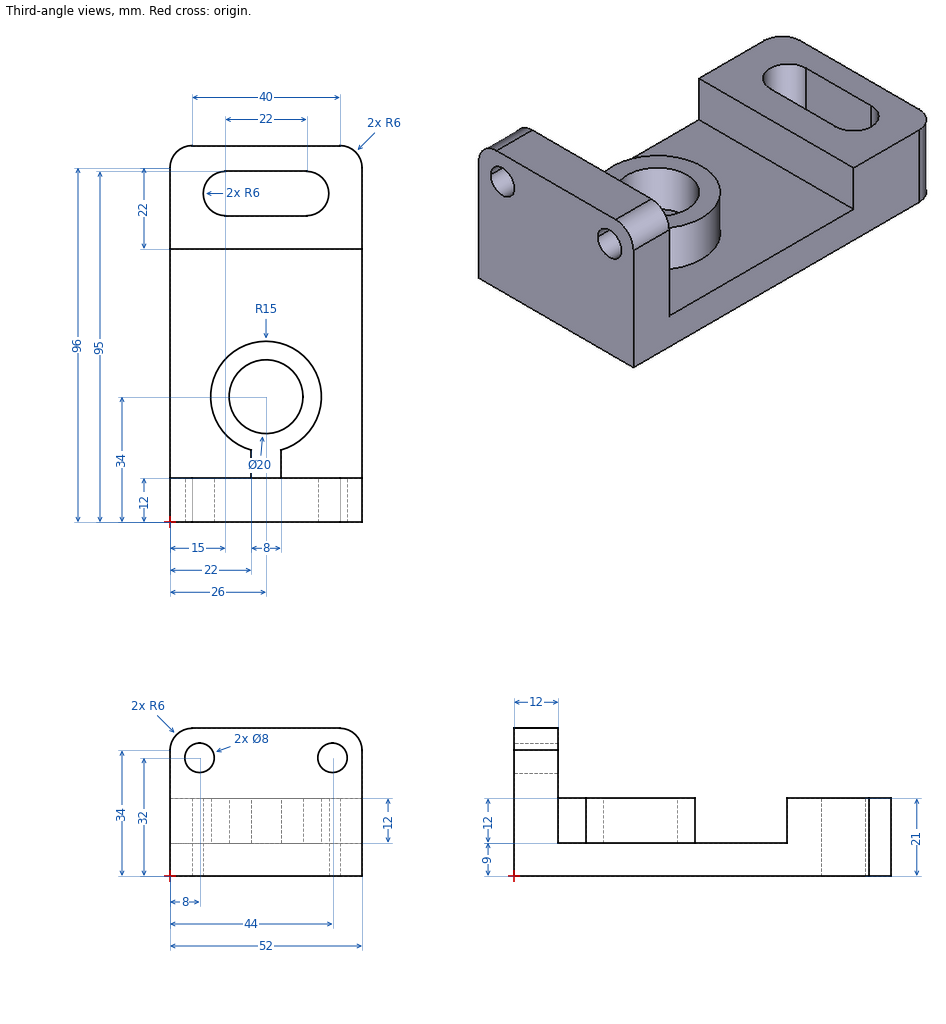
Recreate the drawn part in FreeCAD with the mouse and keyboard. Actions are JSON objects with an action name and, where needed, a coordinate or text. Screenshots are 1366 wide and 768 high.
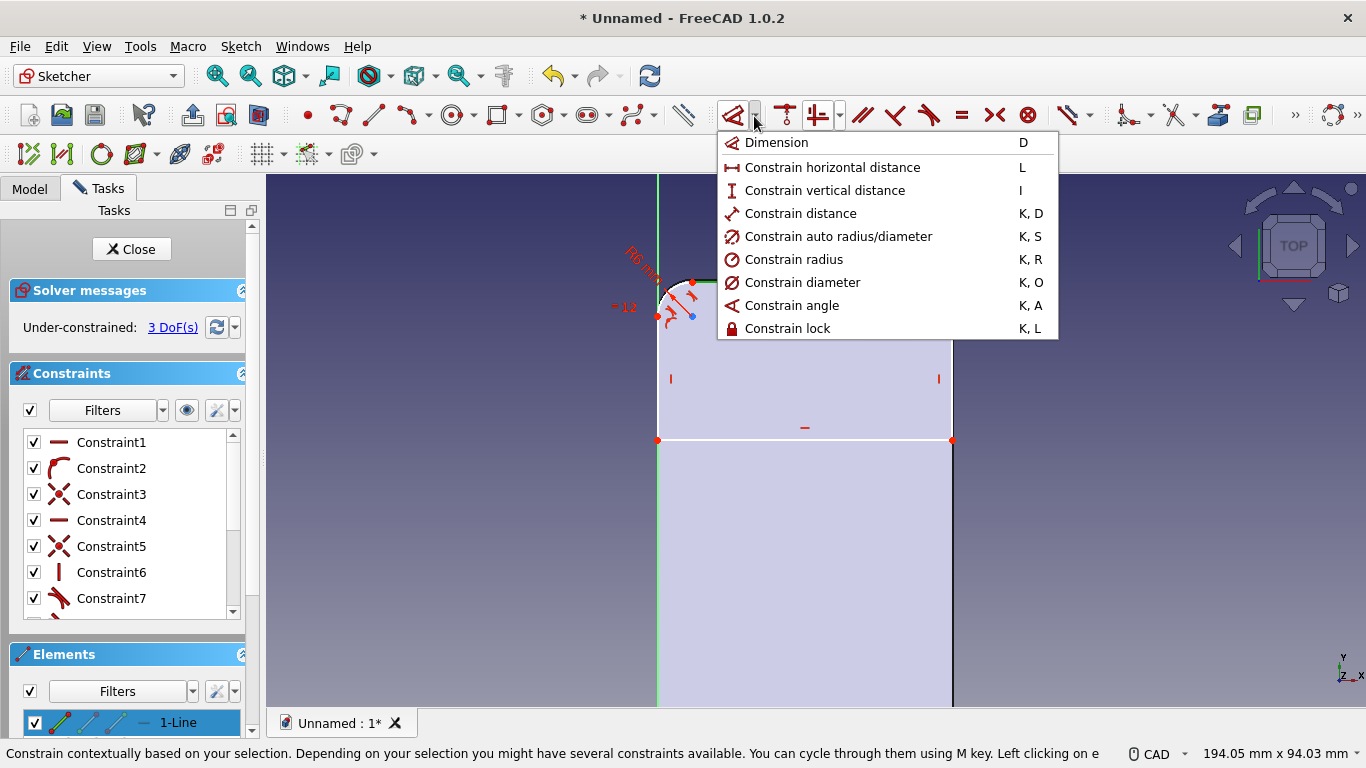
{"action": "left_click", "coordinate": [888, 168]}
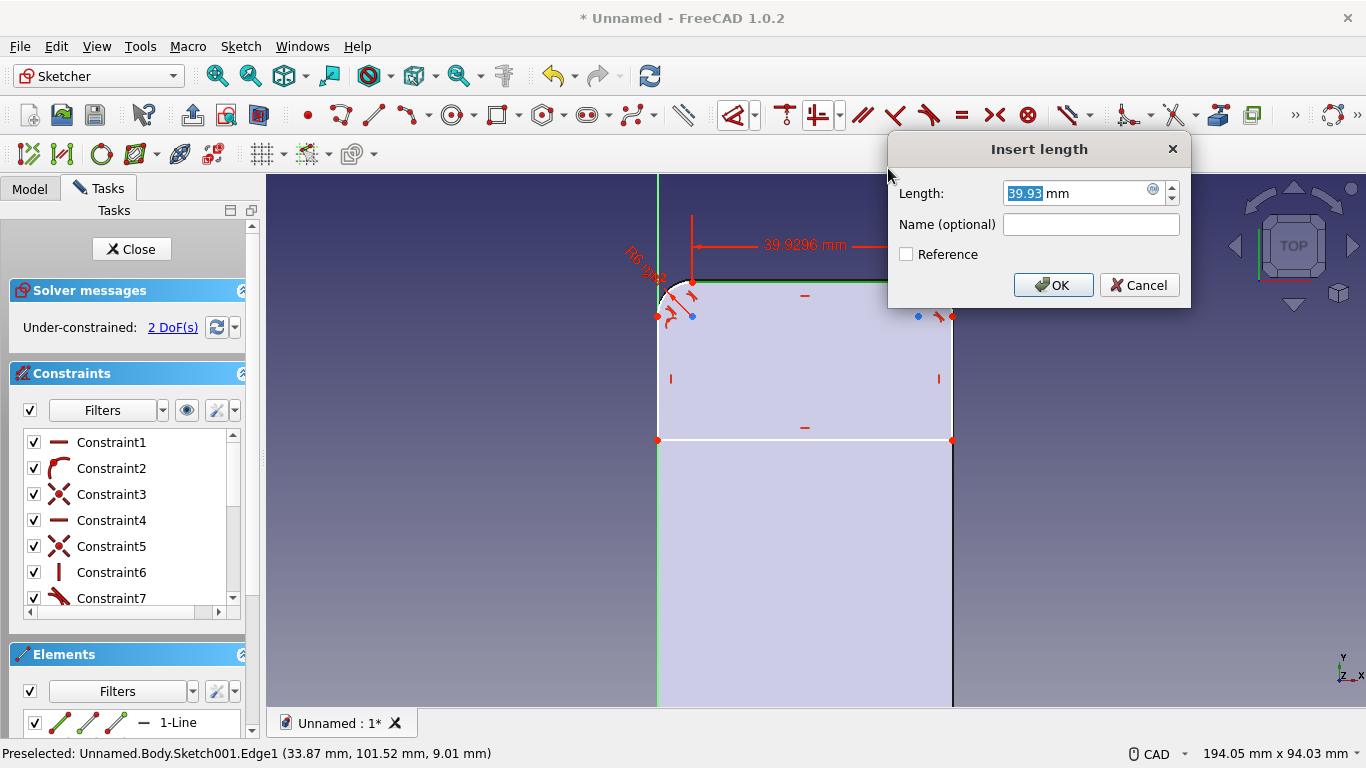
{"action": "type", "text": "40"}
{"action": "key", "text": "Return"}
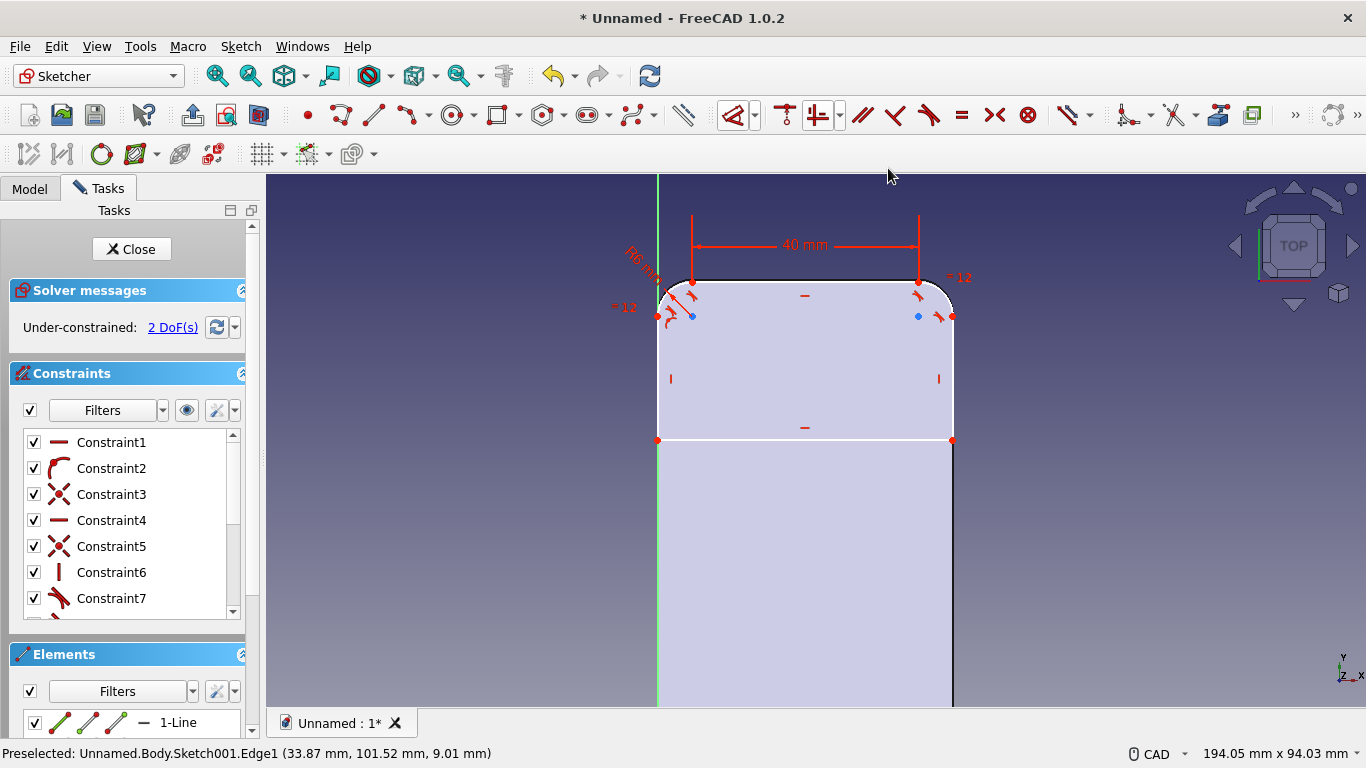
{"action": "left_click", "coordinate": [658, 354]}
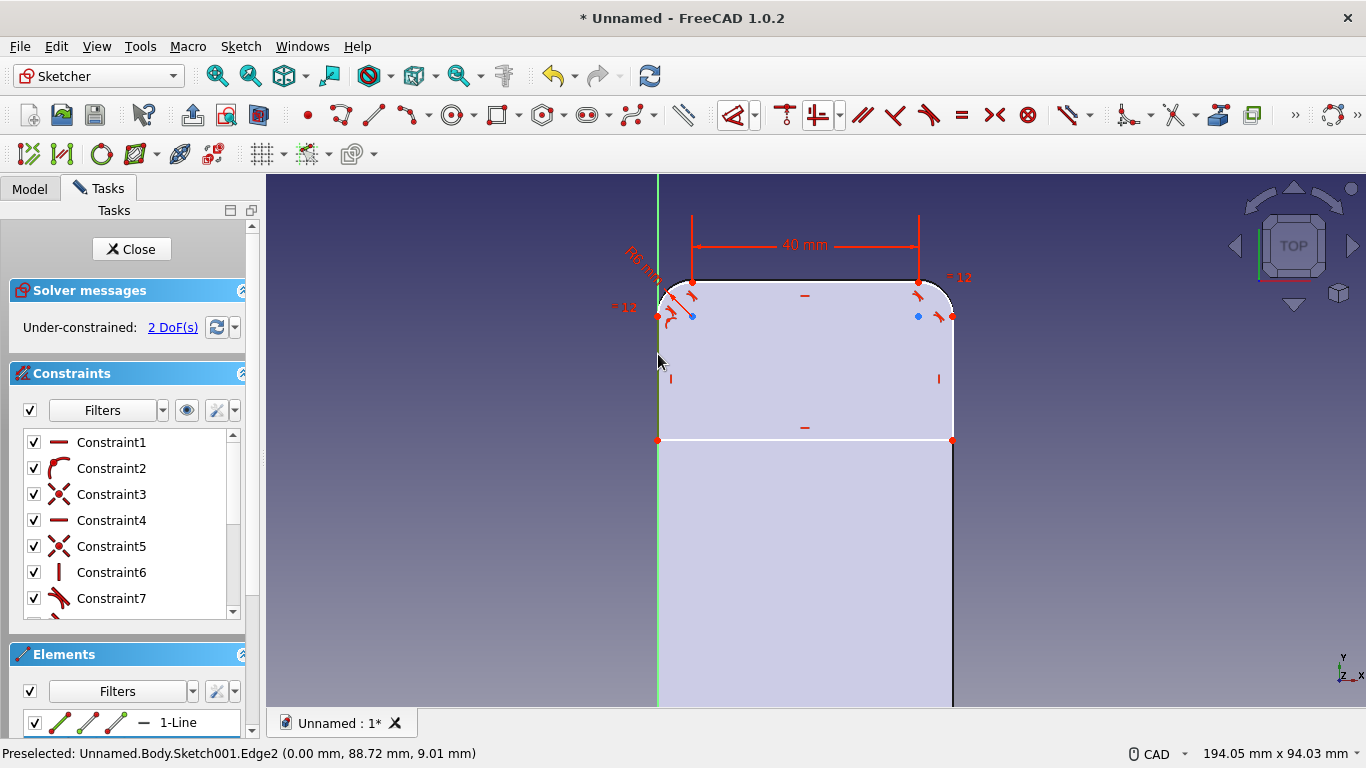
{"action": "key", "text": "i"}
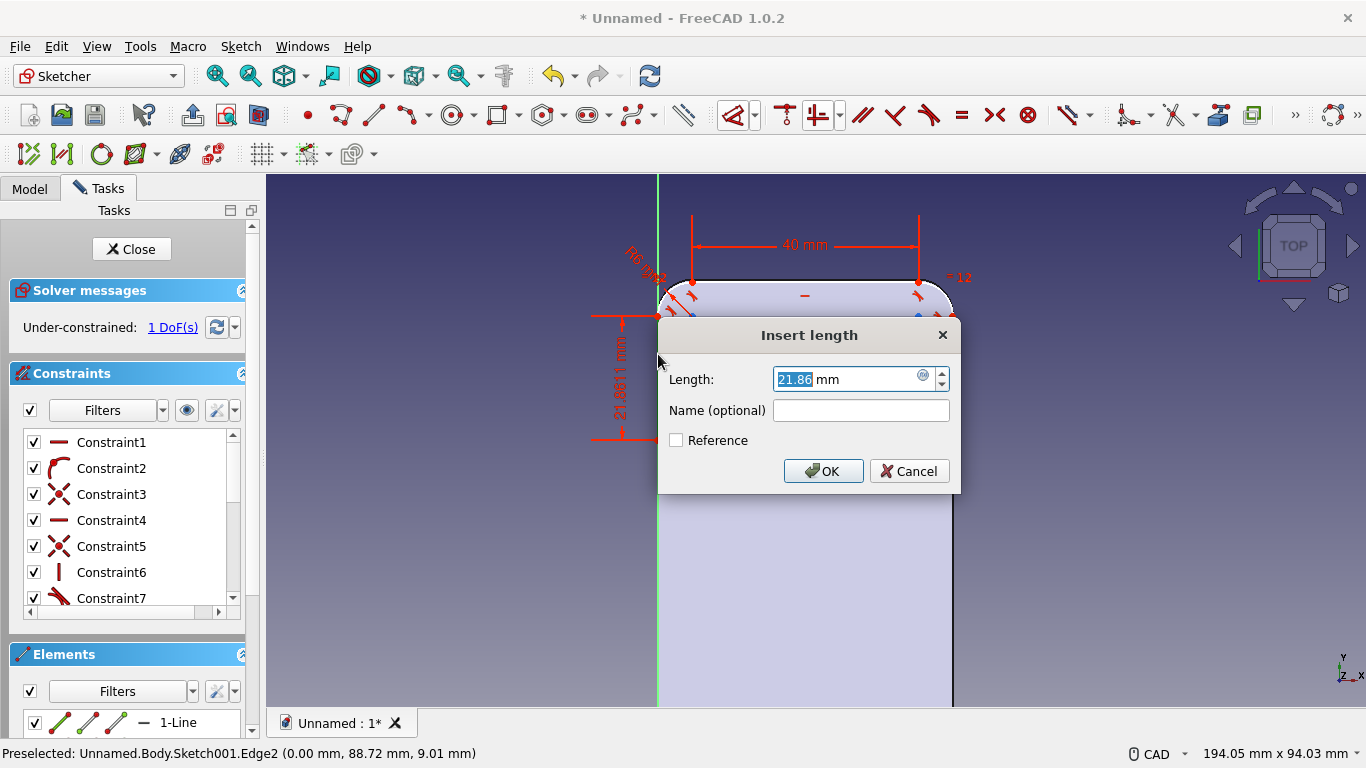
{"action": "type", "text": "22"}
{"action": "key", "text": "Return"}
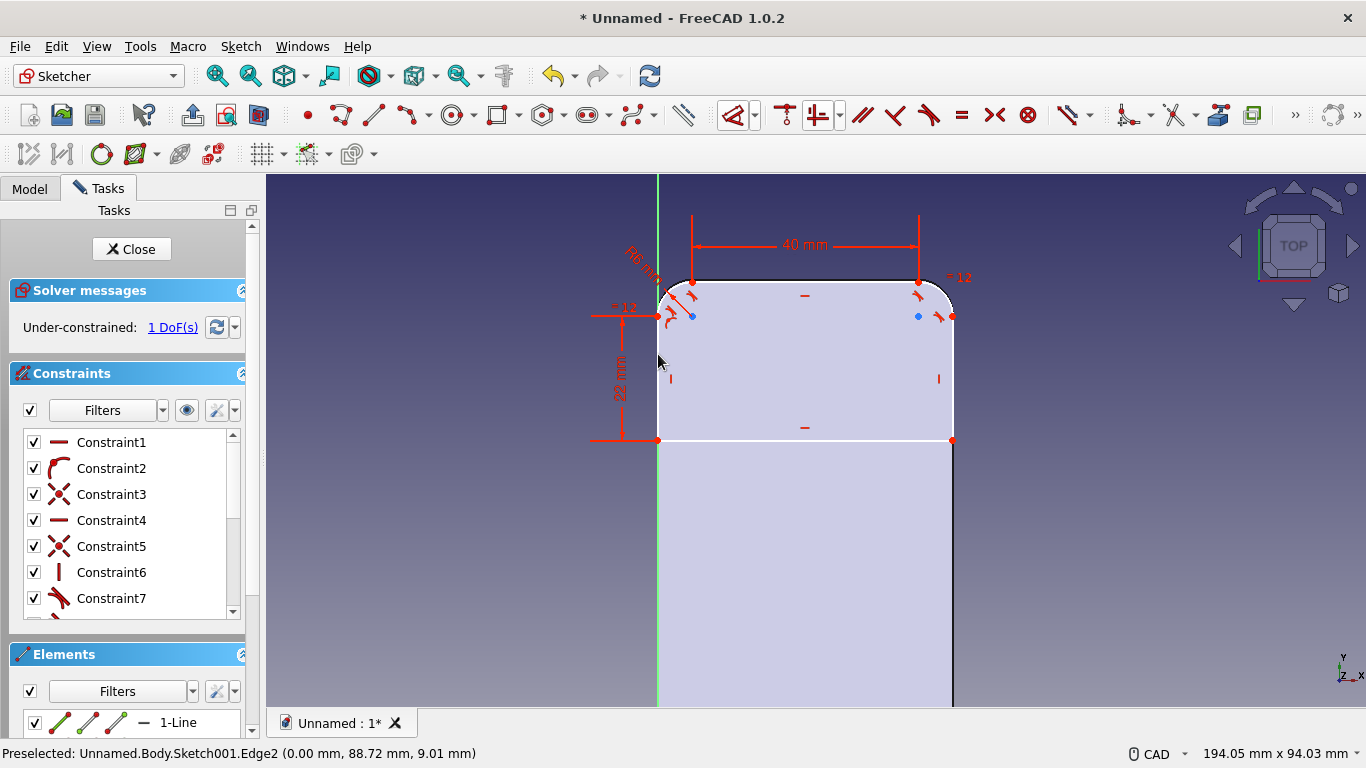
{"action": "left_click", "coordinate": [658, 316]}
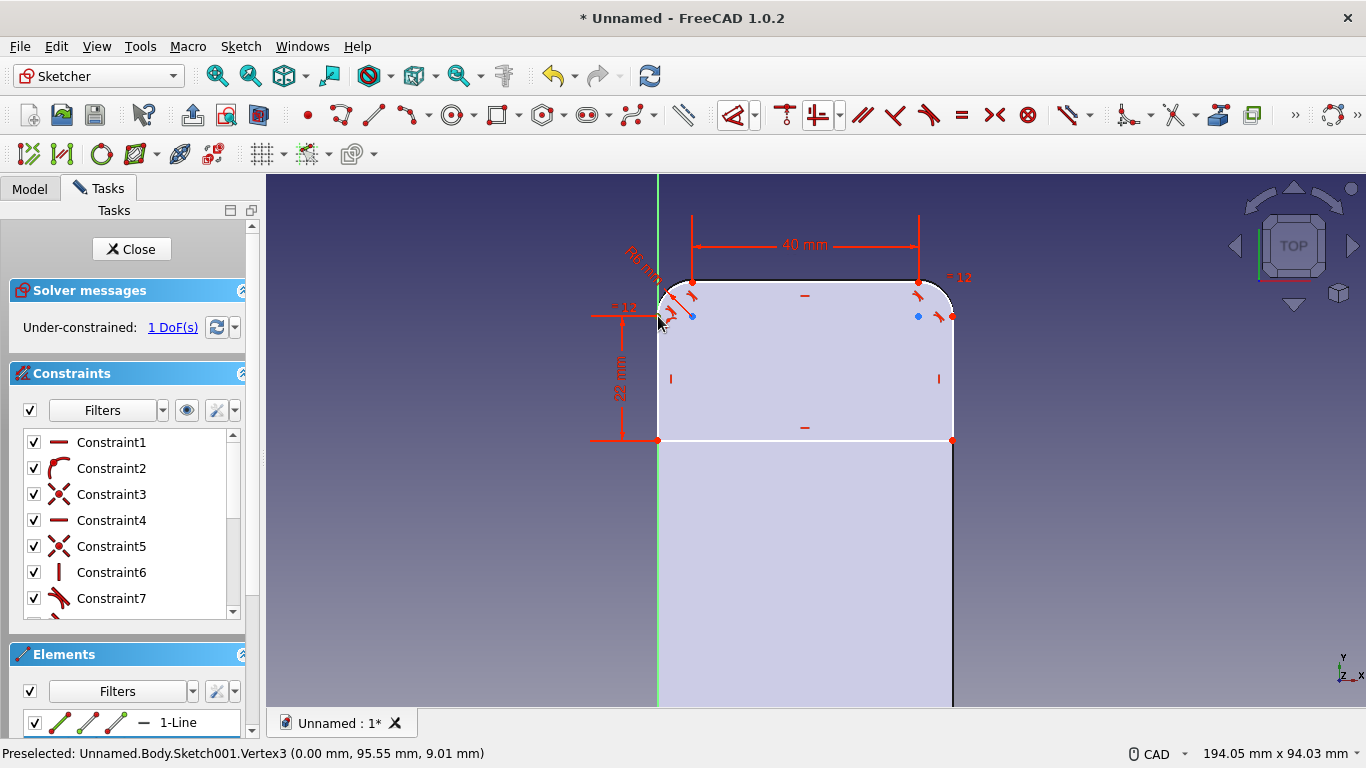
{"action": "key", "text": "i"}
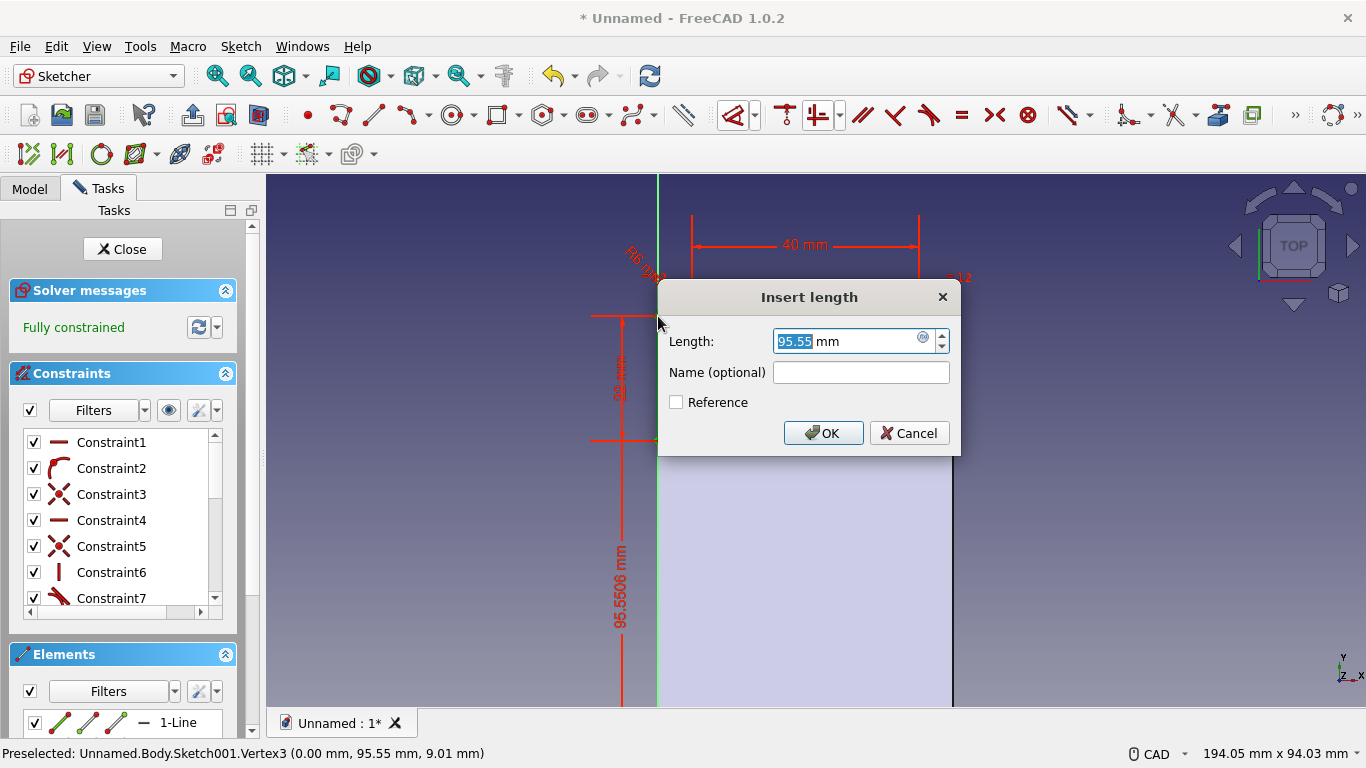
{"action": "type", "text": "96"}
{"action": "key", "text": "Return"}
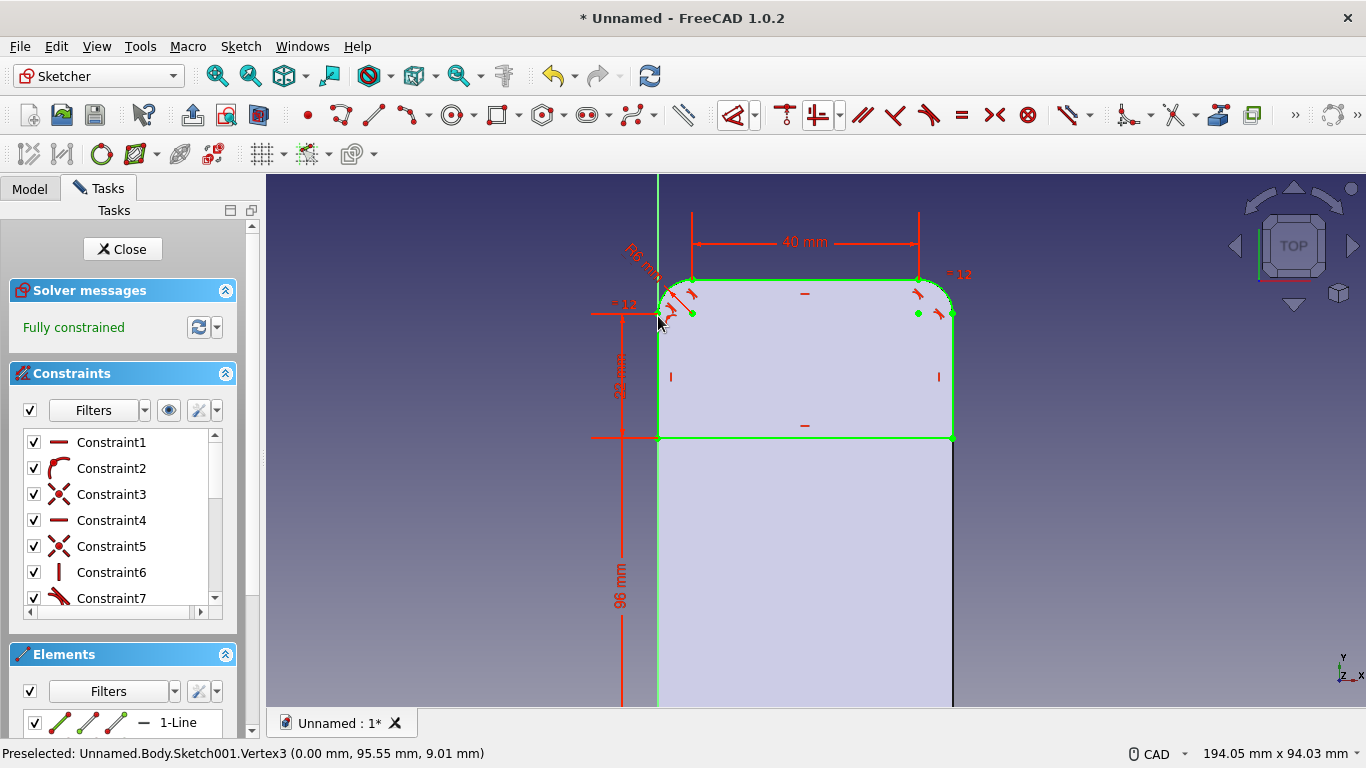
{"action": "left_click", "coordinate": [123, 249]}